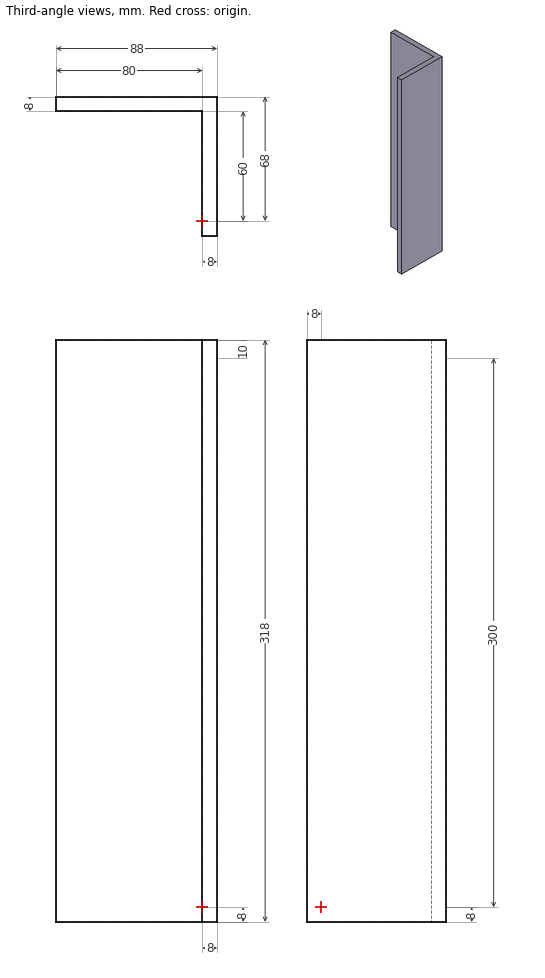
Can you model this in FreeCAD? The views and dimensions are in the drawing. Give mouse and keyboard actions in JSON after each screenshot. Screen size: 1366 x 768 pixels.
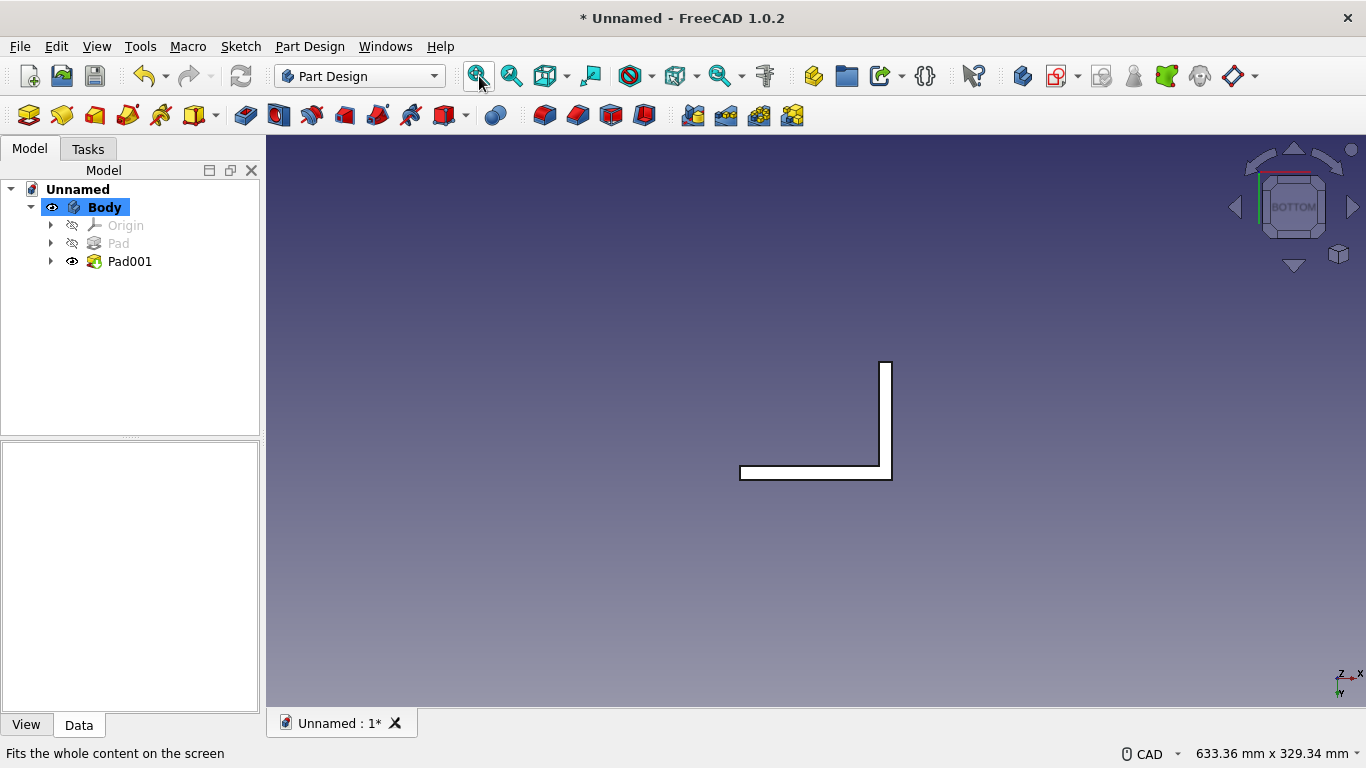
{"action": "key", "text": "v f"}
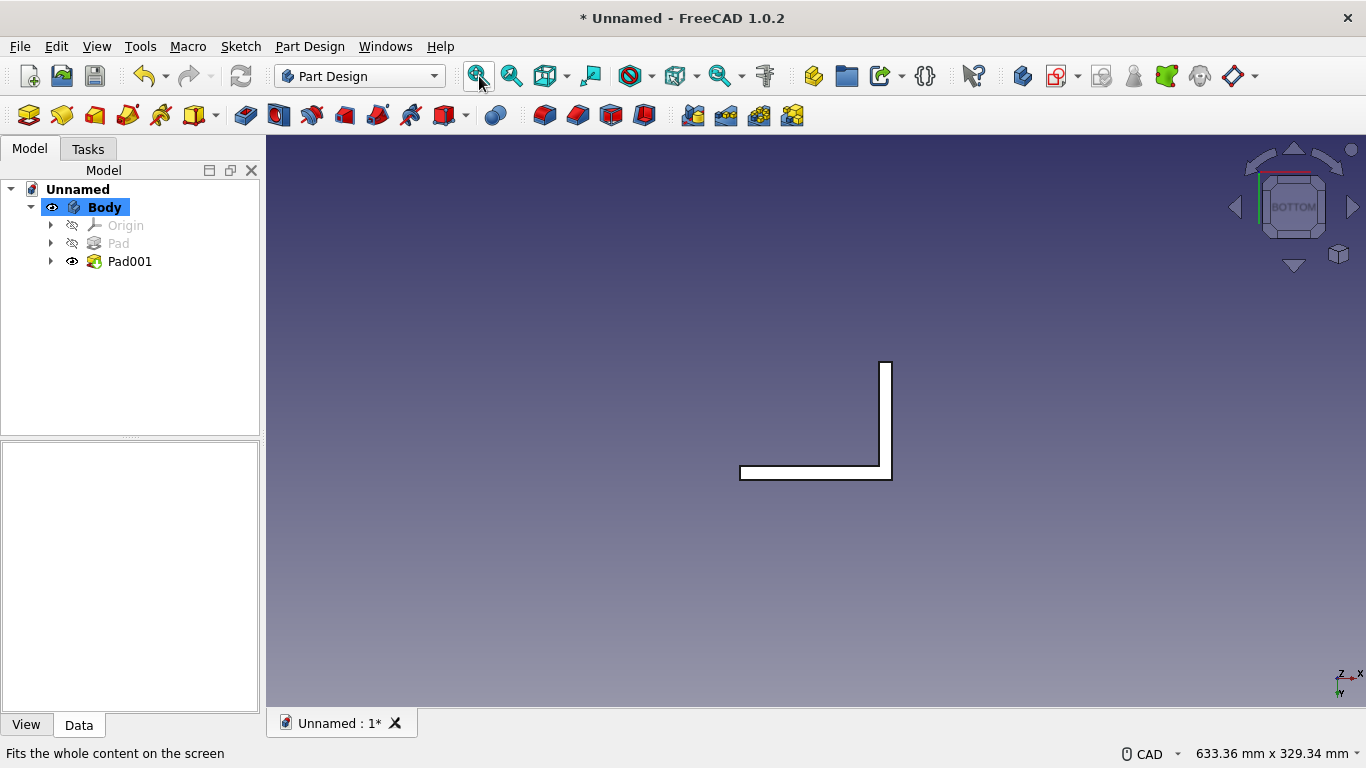
{"action": "scroll", "coordinate": [882, 471], "scroll_direction": "up", "scroll_amount": 4}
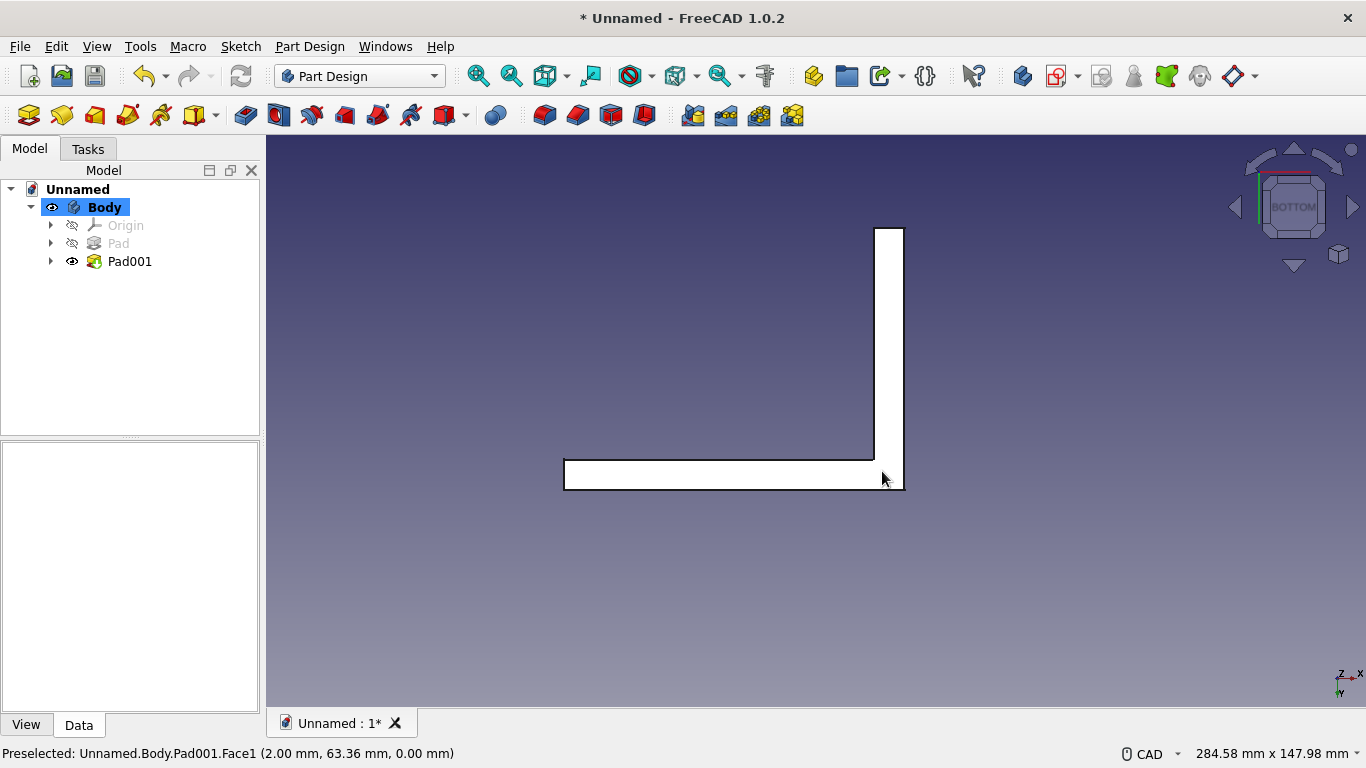
{"action": "left_click", "coordinate": [880, 471]}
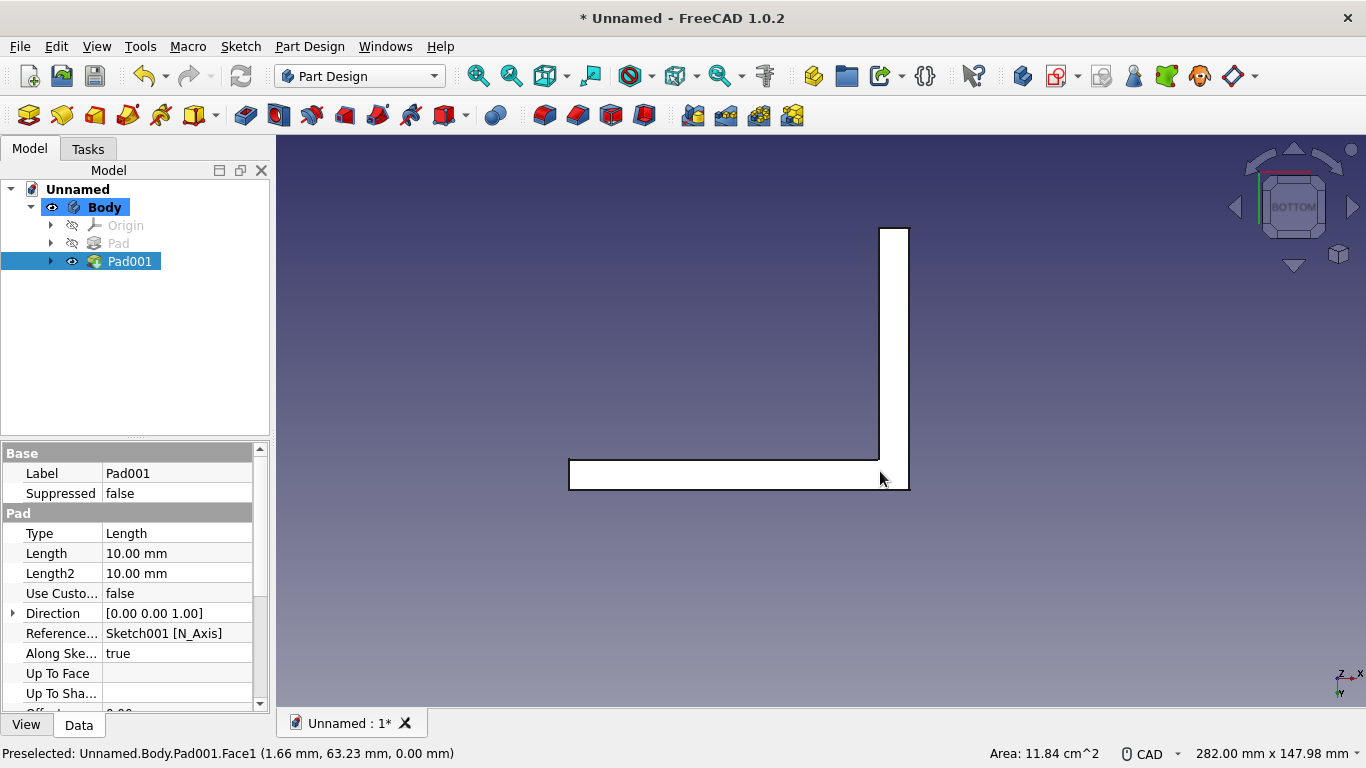
{"action": "left_click", "coordinate": [1056, 76]}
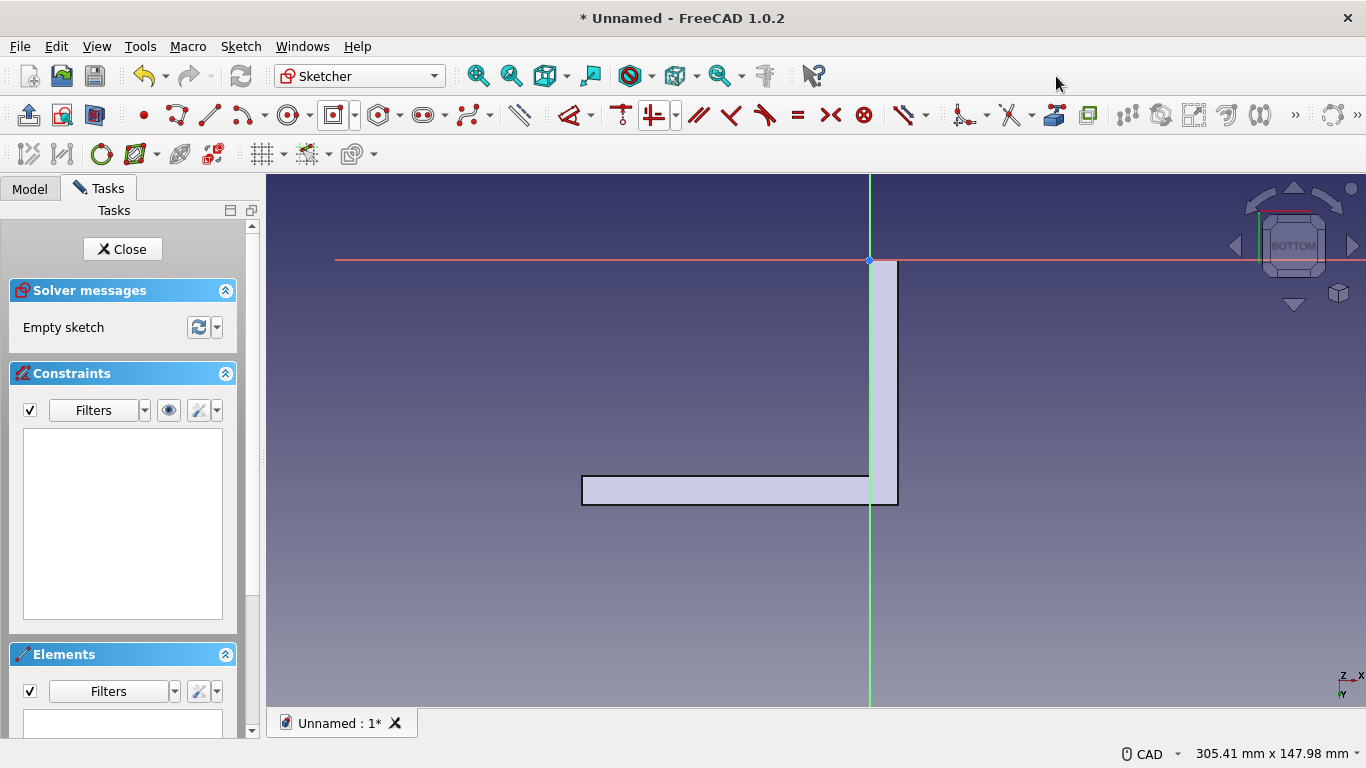
{"action": "scroll", "coordinate": [725, 265], "scroll_direction": "up", "scroll_amount": 2}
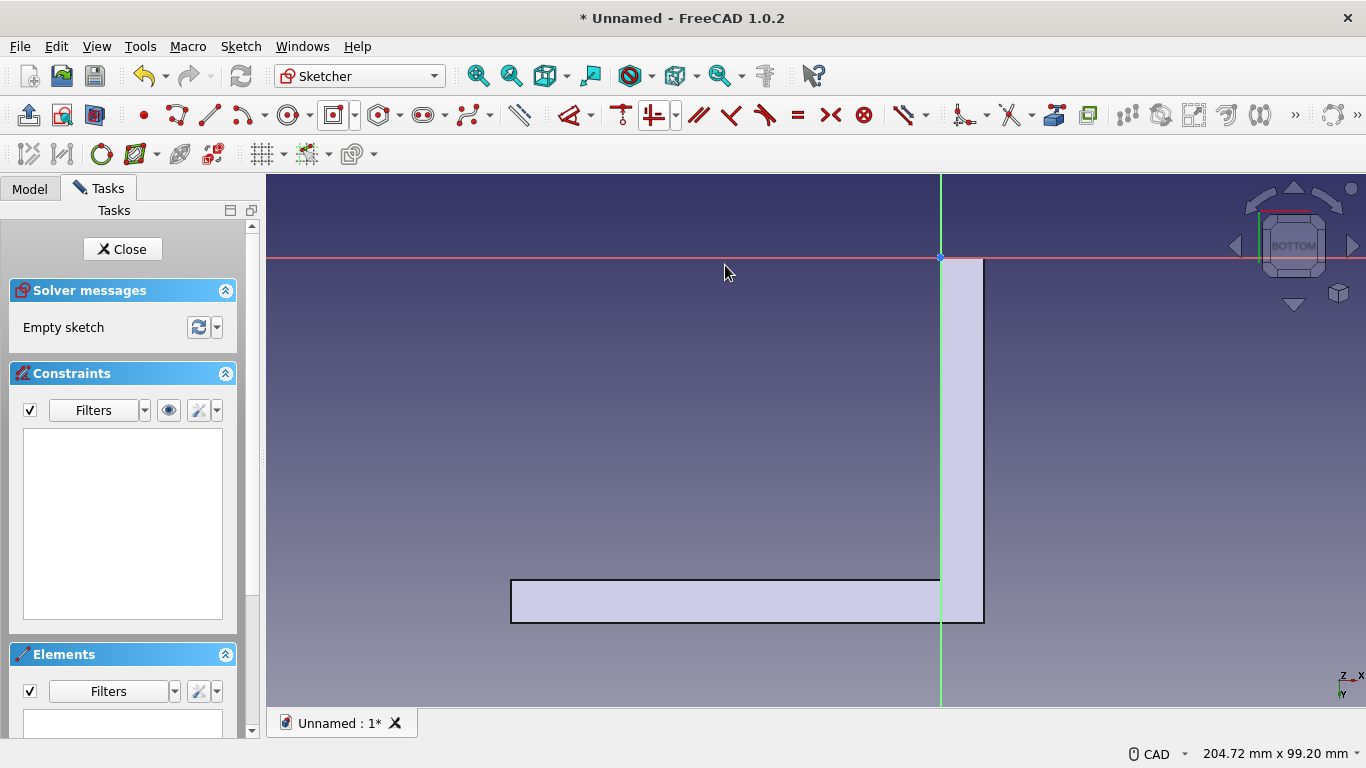
{"action": "left_click", "coordinate": [177, 116]}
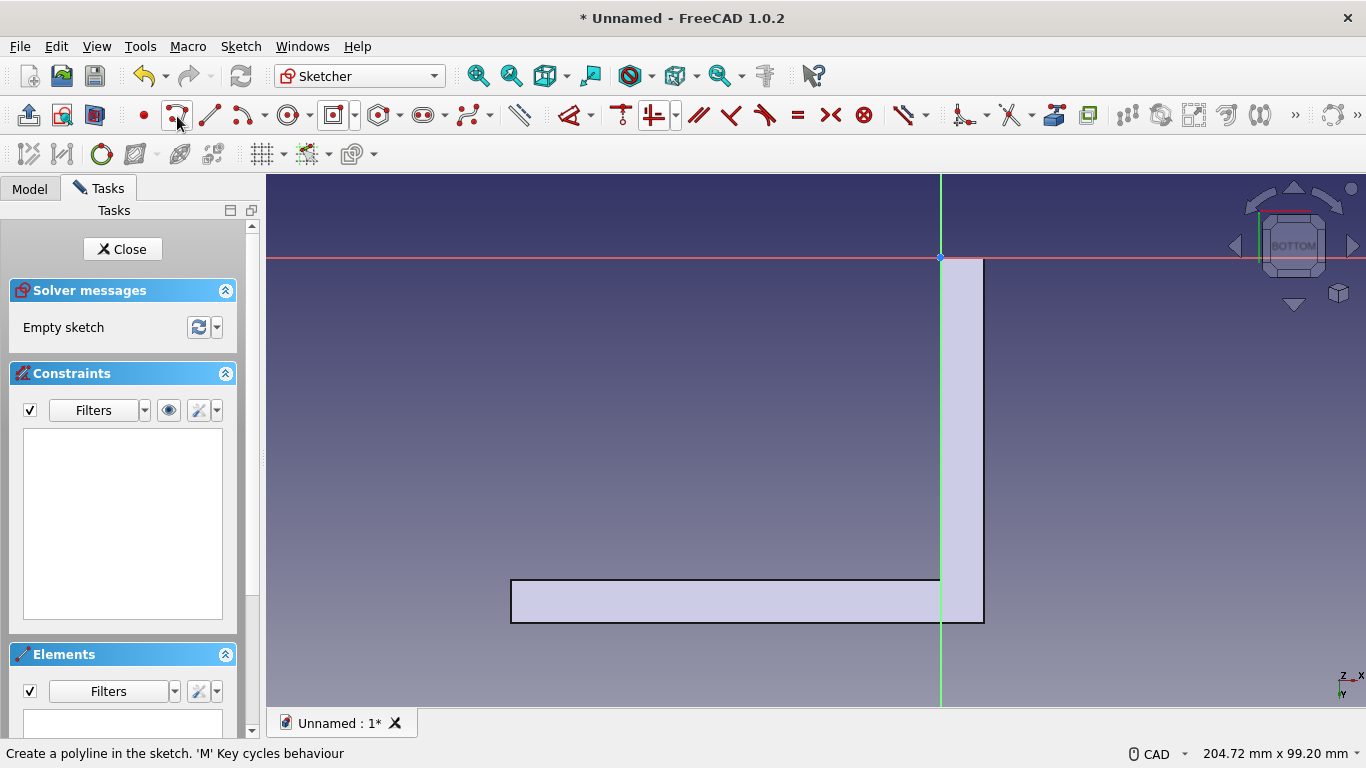
{"action": "left_click", "coordinate": [941, 258]}
{"action": "left_click", "coordinate": [932, 580]}
{"action": "left_click", "coordinate": [511, 580]}
{"action": "left_click", "coordinate": [511, 623]}
{"action": "left_click", "coordinate": [984, 623]}
{"action": "left_click", "coordinate": [984, 267]}
{"action": "left_click", "coordinate": [941, 258]}
{"action": "key", "text": "Escape"}
{"action": "key", "text": "Escape"}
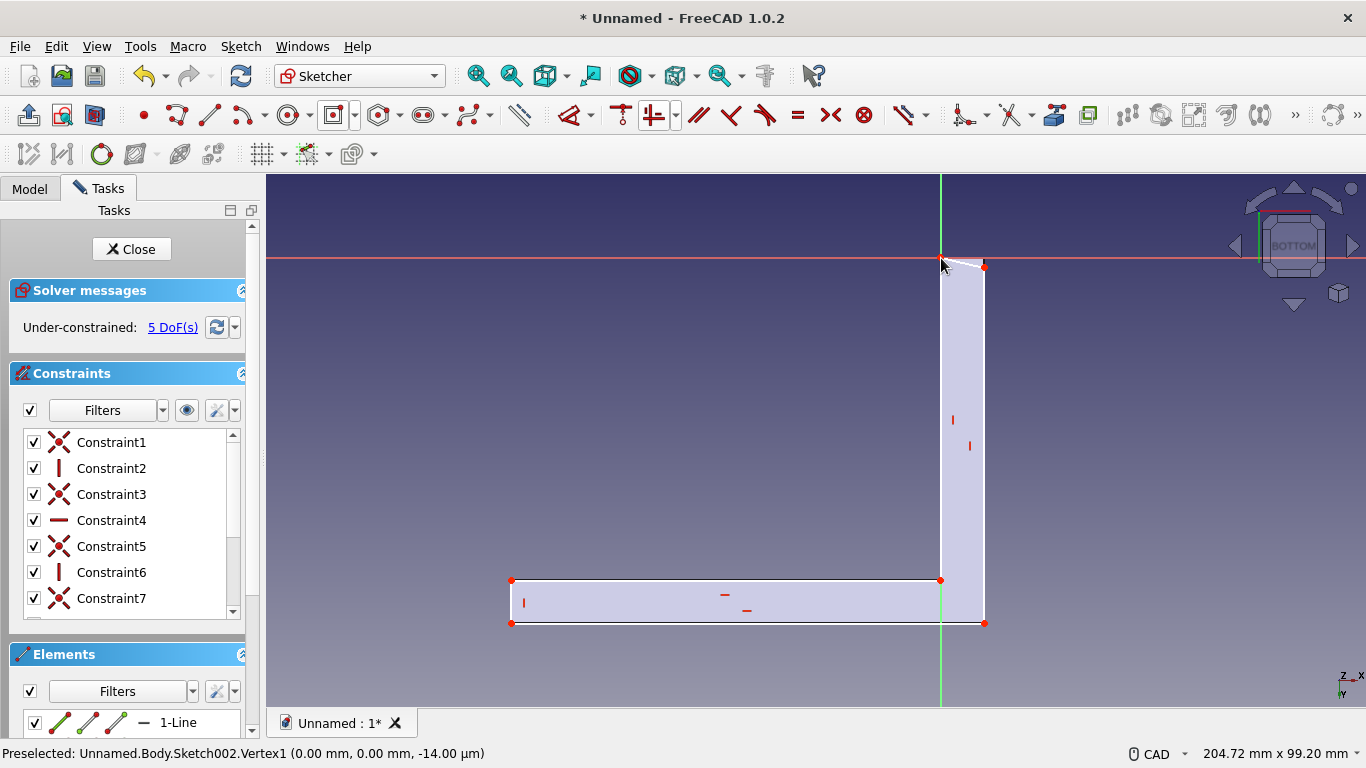
{"action": "left_click", "coordinate": [954, 261]}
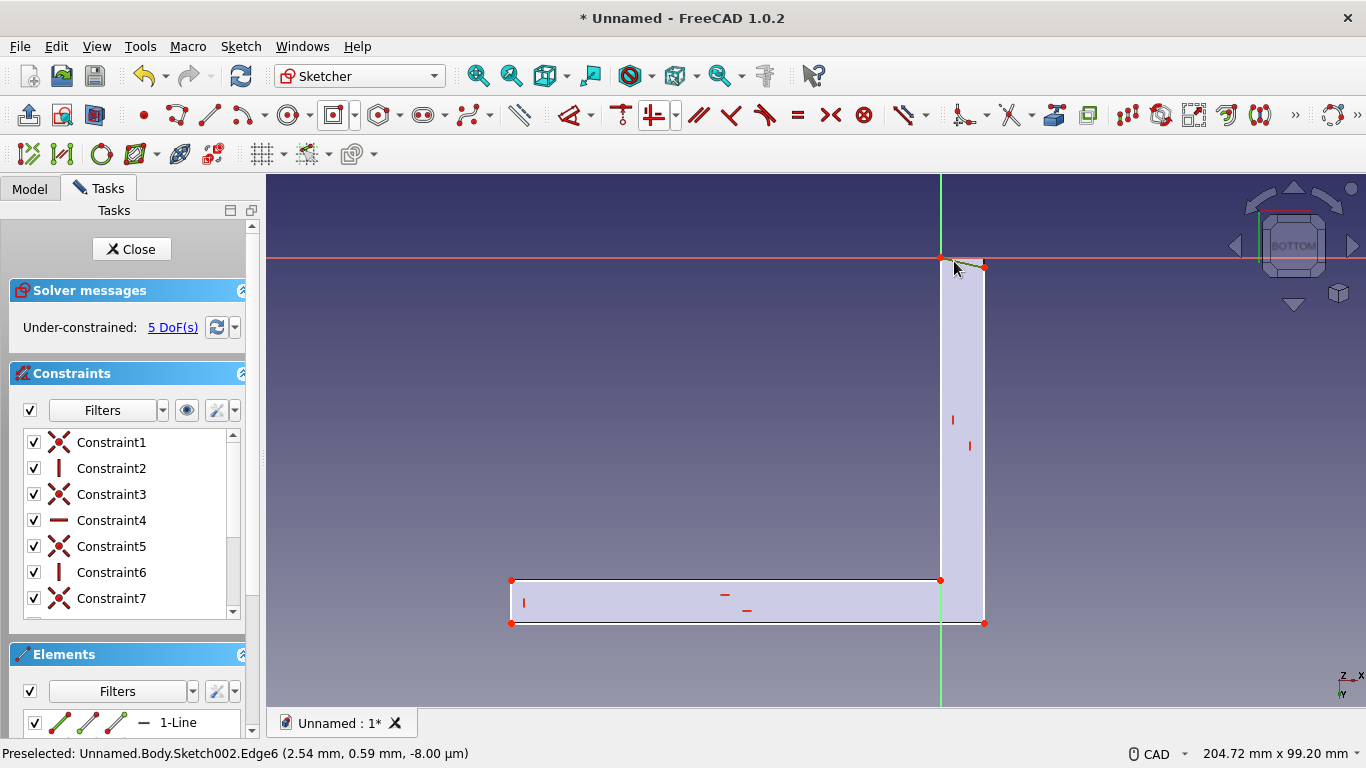
{"action": "left_click", "coordinate": [676, 116]}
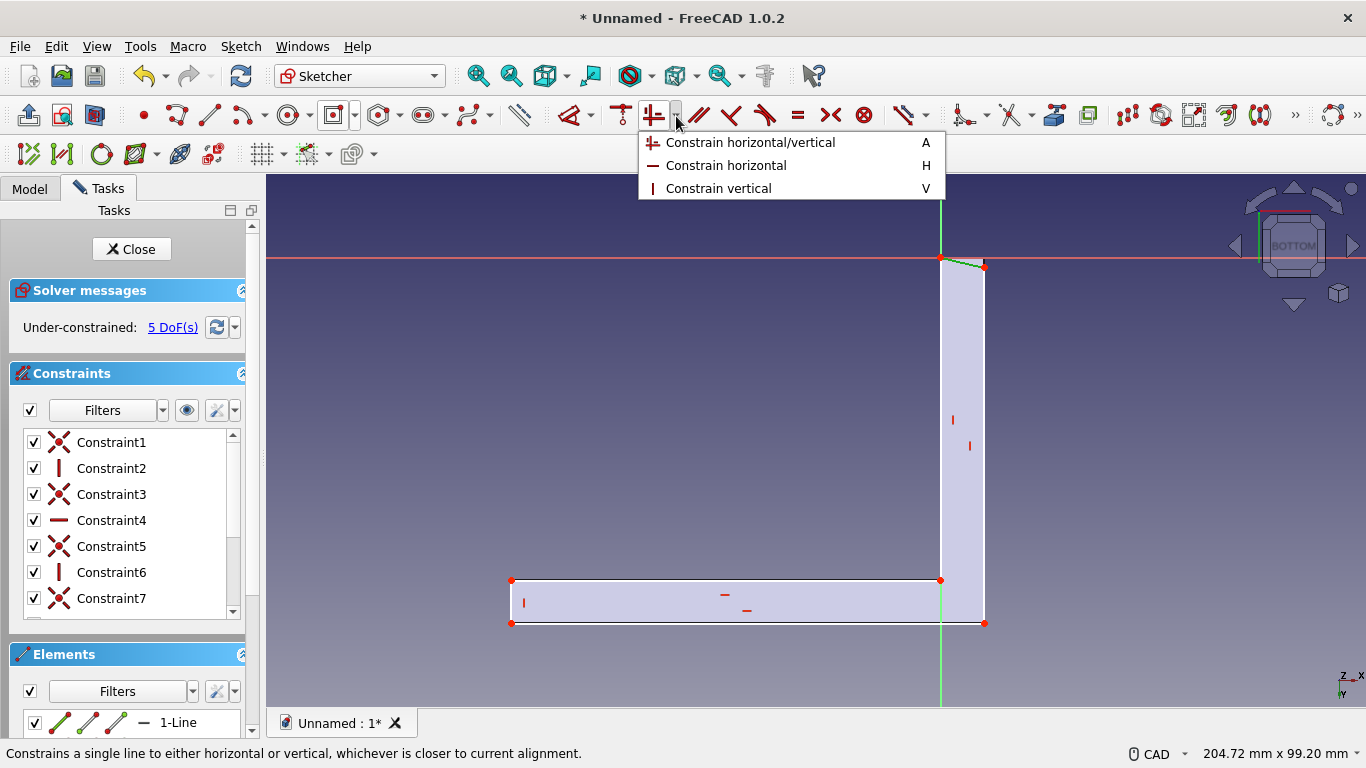
{"action": "left_click", "coordinate": [792, 166]}